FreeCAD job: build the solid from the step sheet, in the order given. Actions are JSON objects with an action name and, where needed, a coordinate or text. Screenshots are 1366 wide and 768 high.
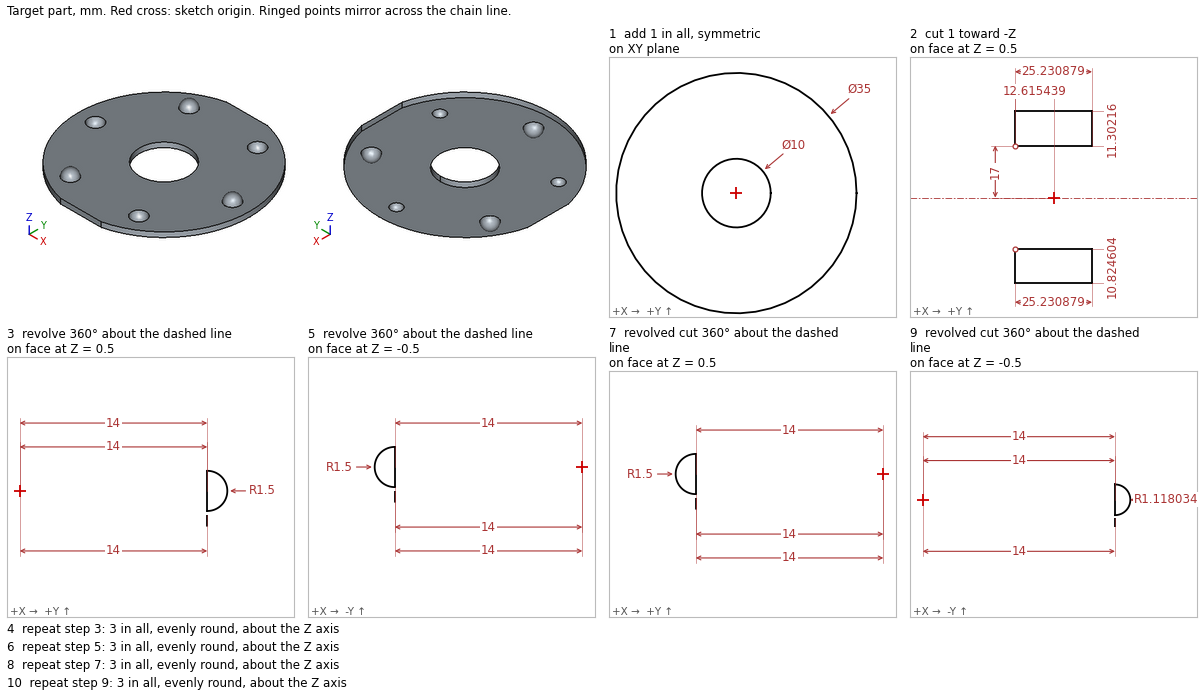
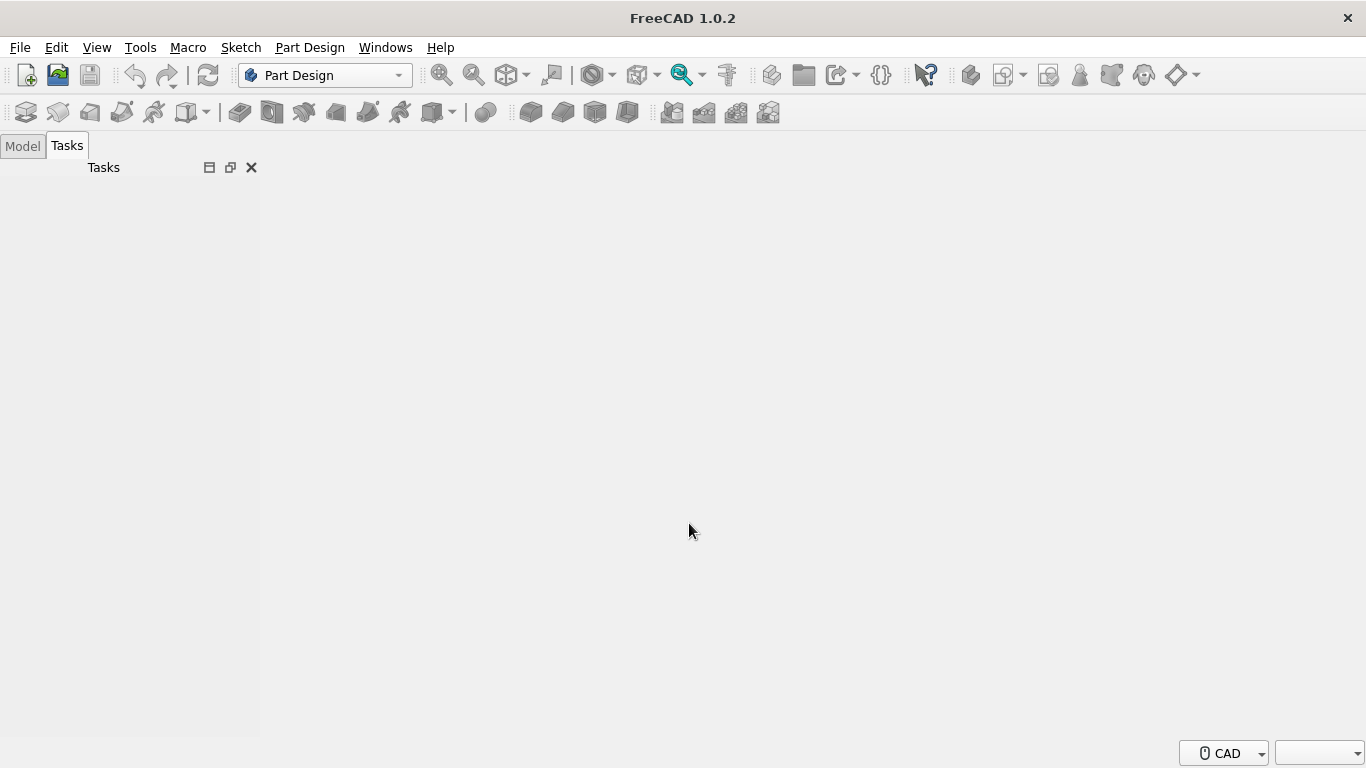
{"action": "key", "text": "ctrl+n"}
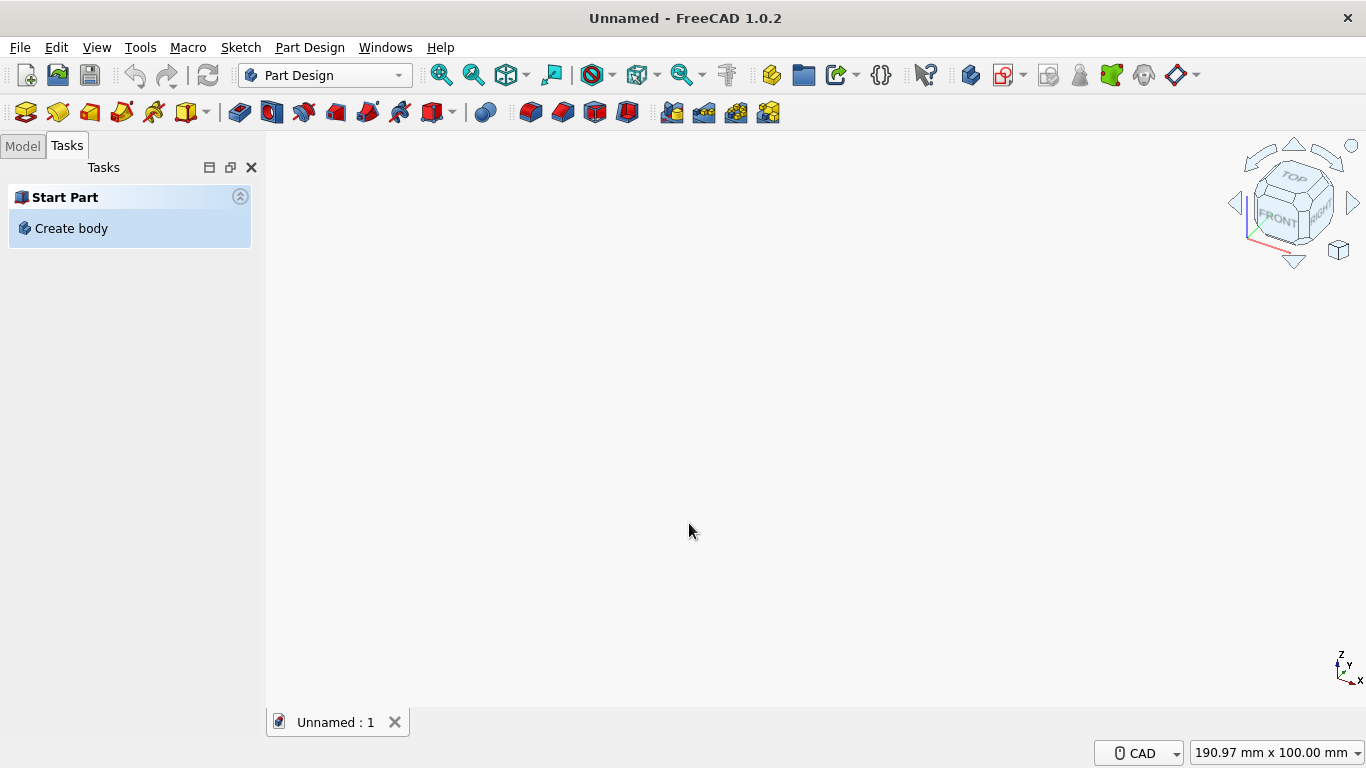
{"action": "left_click", "coordinate": [1004, 76]}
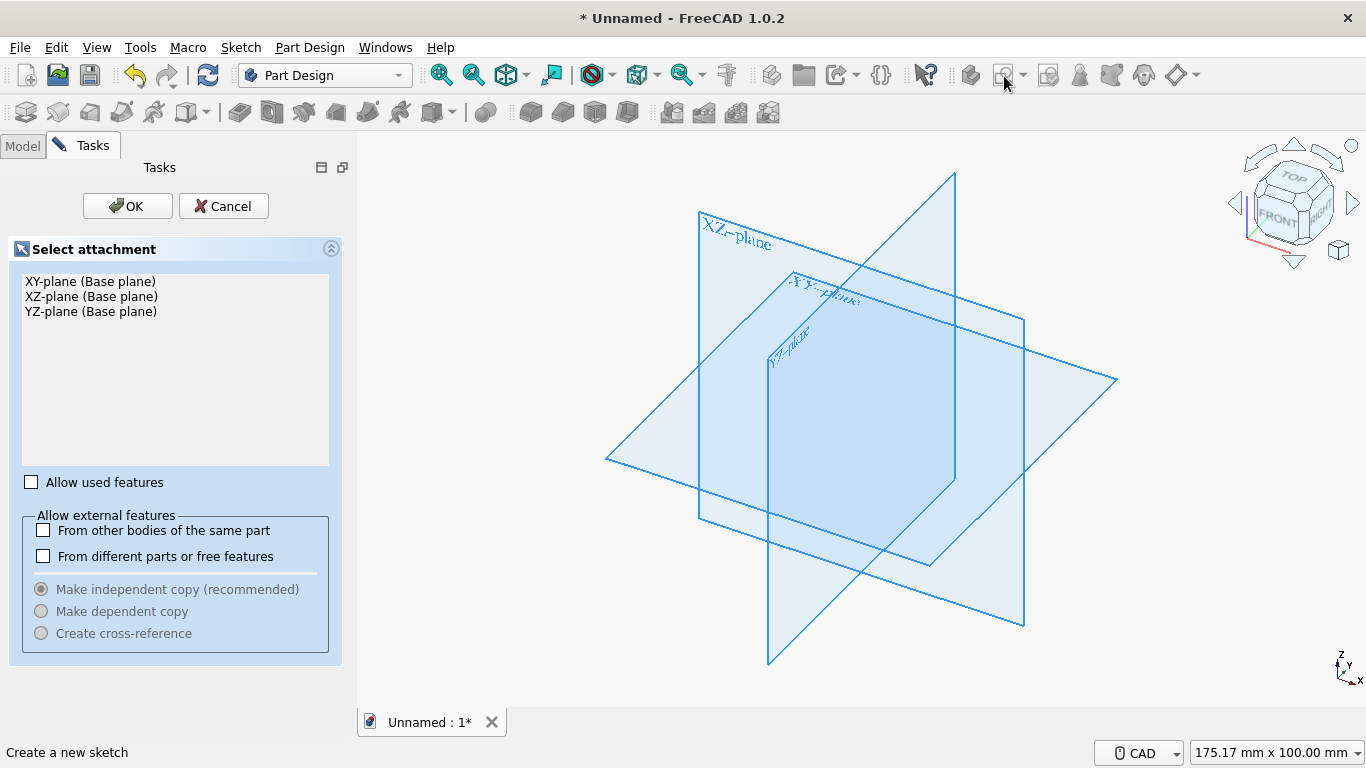
{"action": "left_click", "coordinate": [82, 282]}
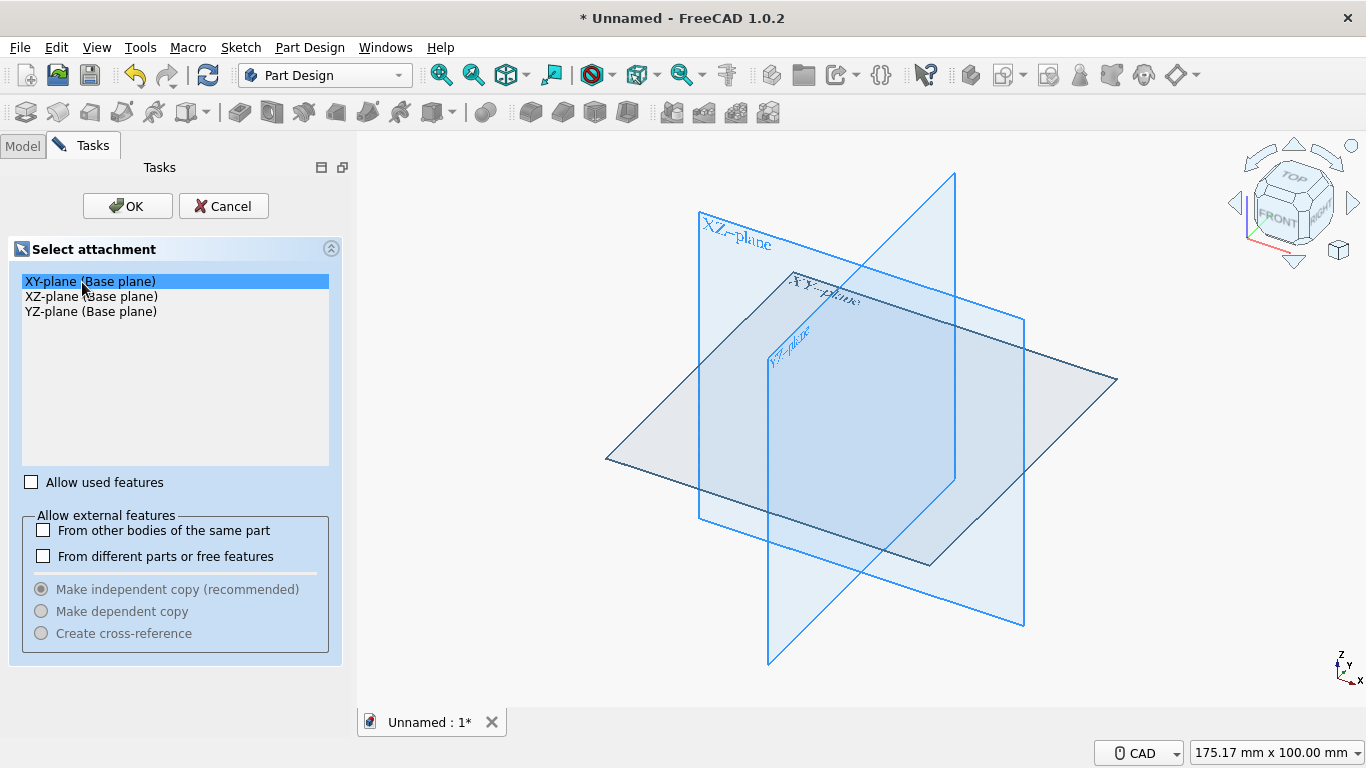
{"action": "left_click", "coordinate": [128, 206]}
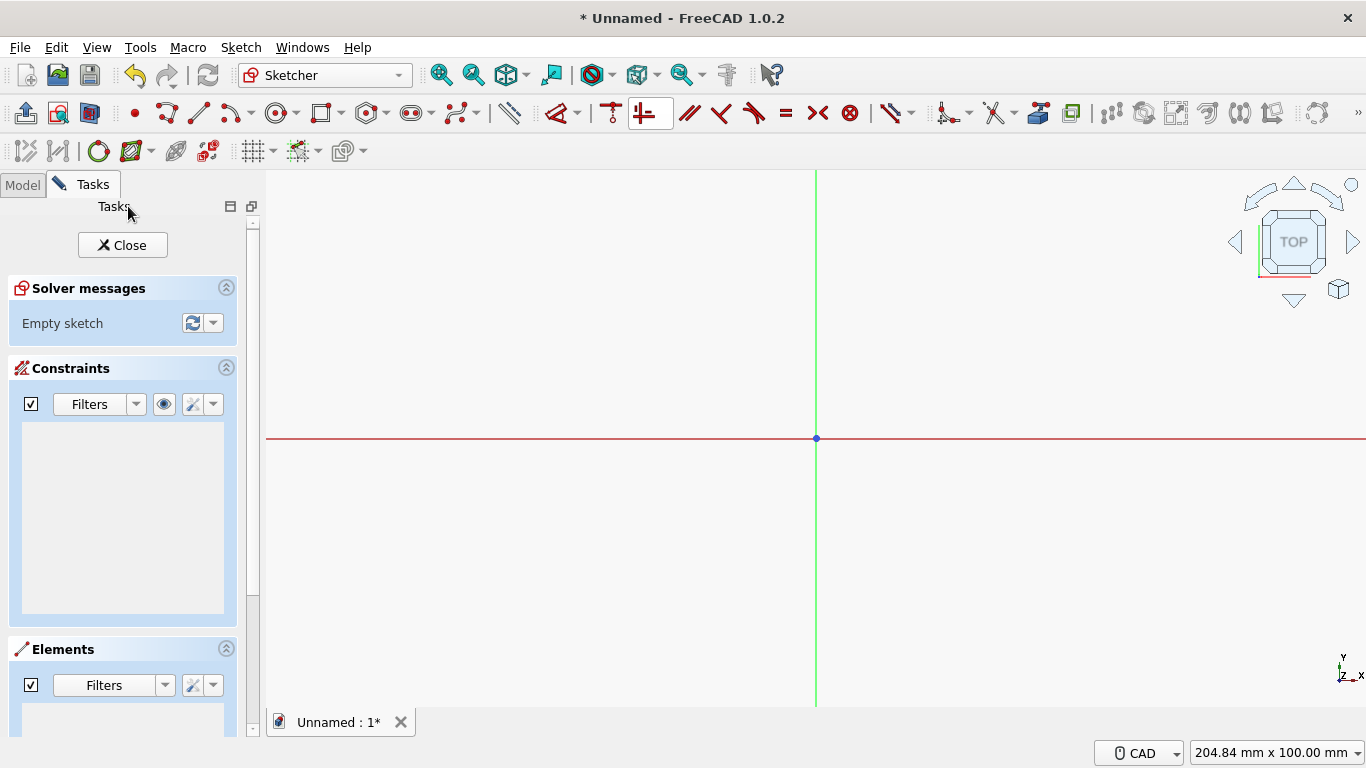
{"action": "scroll", "coordinate": [899, 438], "scroll_direction": "up", "scroll_amount": 3}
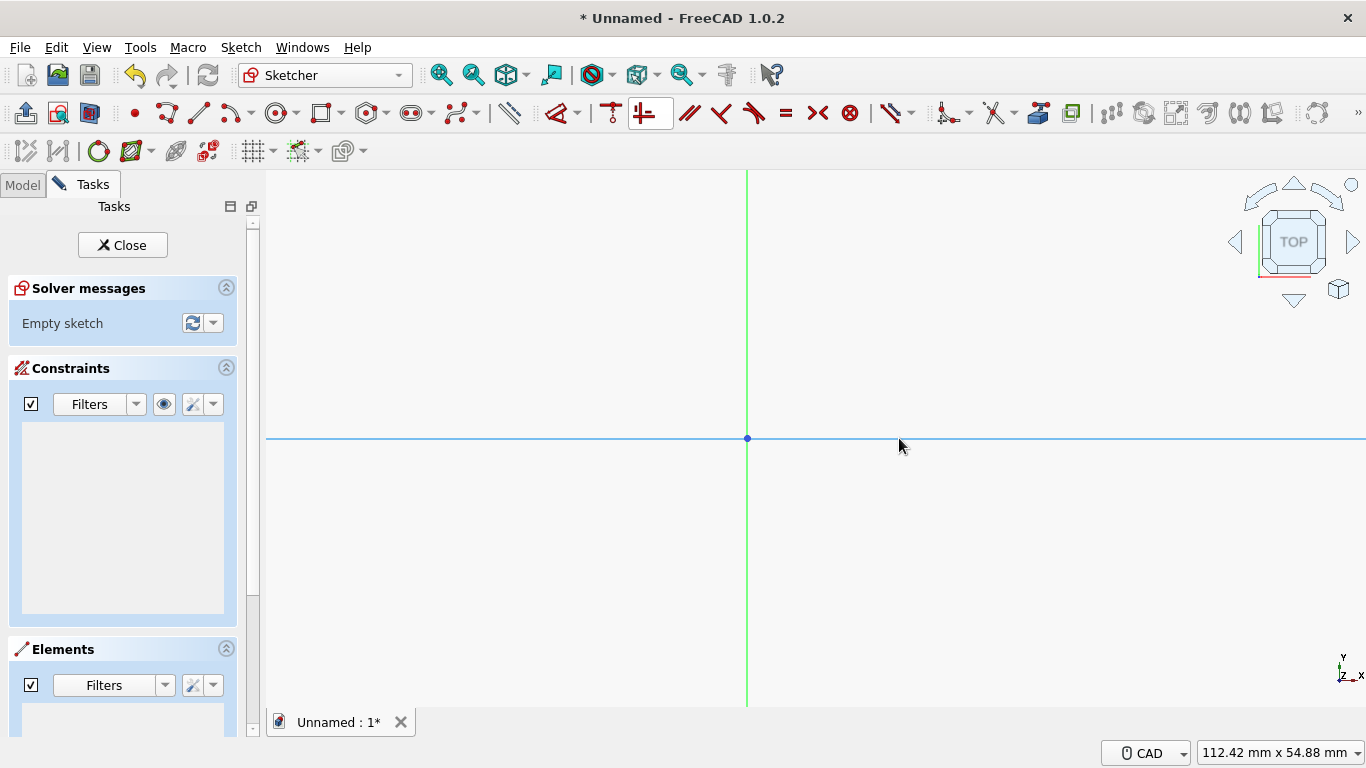
{"action": "key", "text": "g c"}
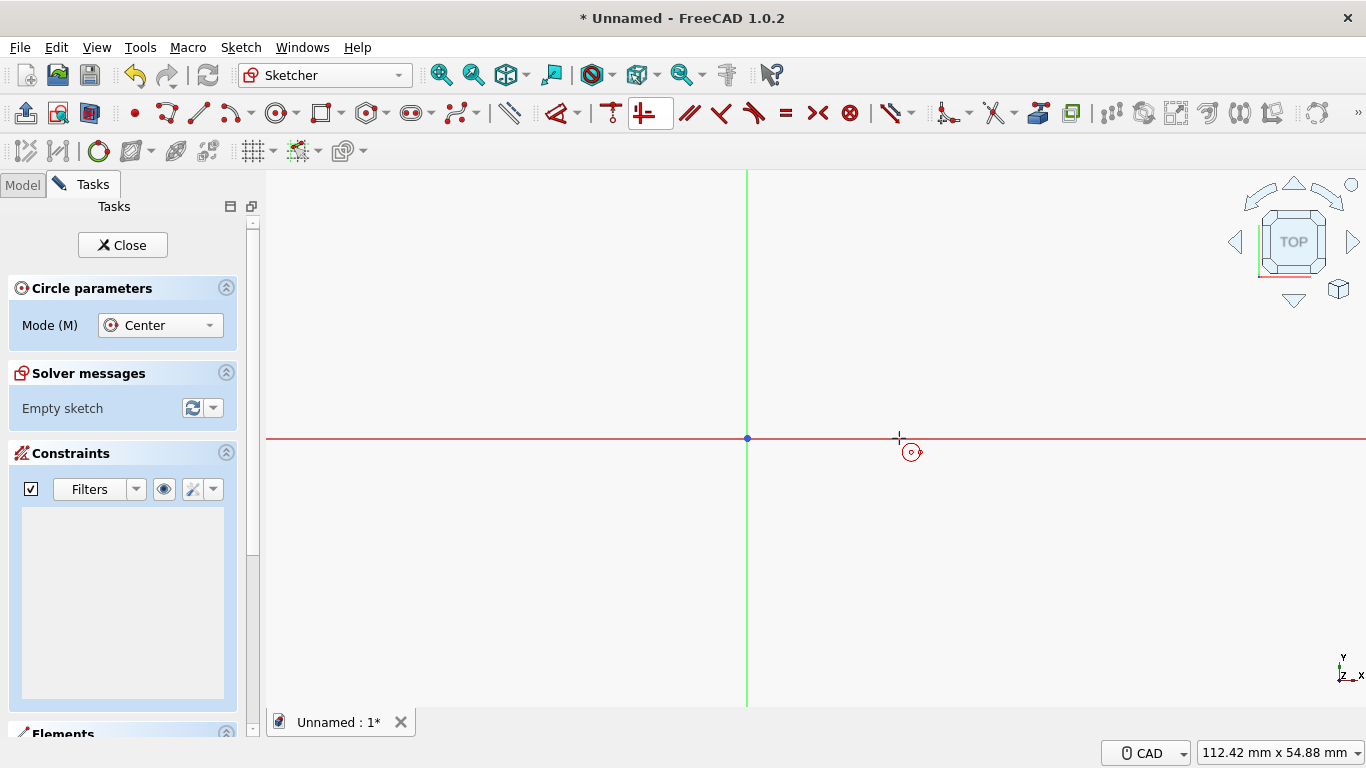
{"action": "left_click", "coordinate": [747, 438]}
{"action": "mouse_move", "coordinate": [868, 317]}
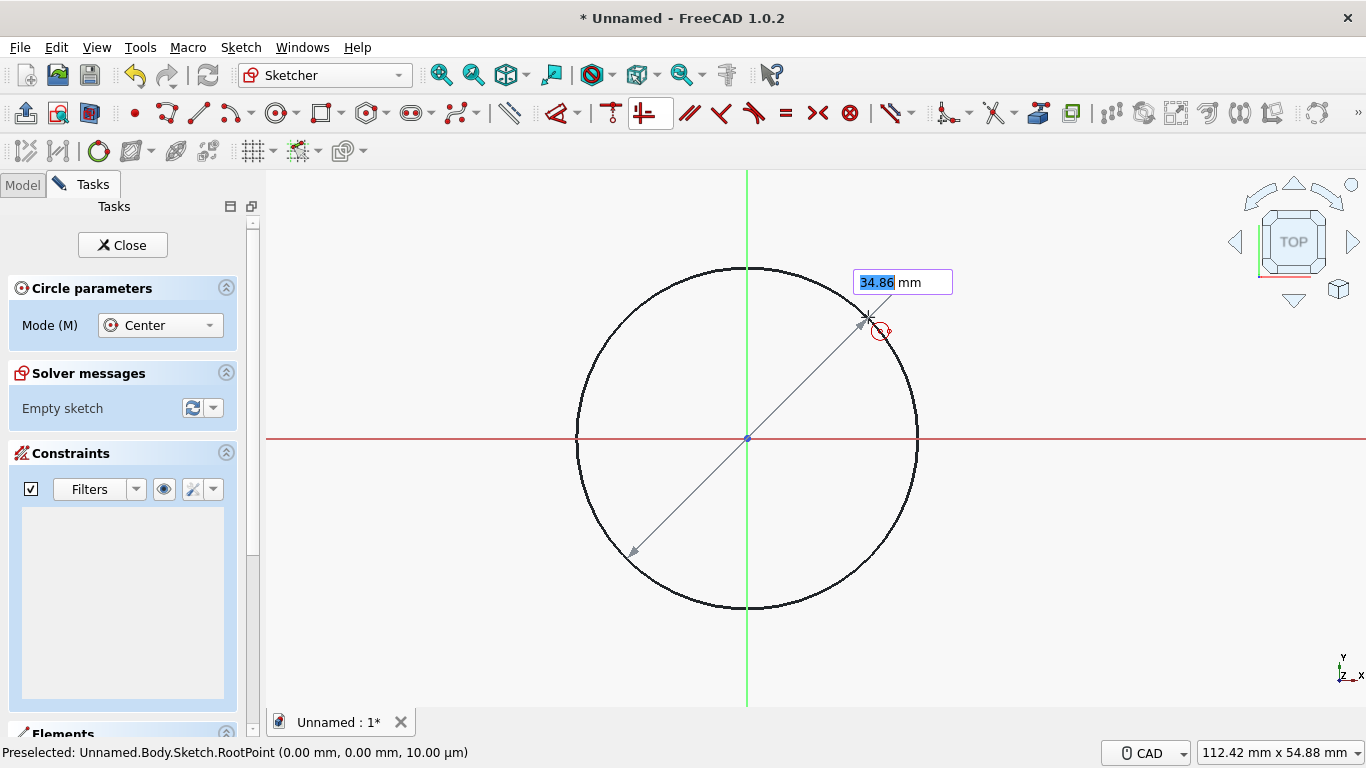
{"action": "type", "text": "35"}
{"action": "key", "text": "Return"}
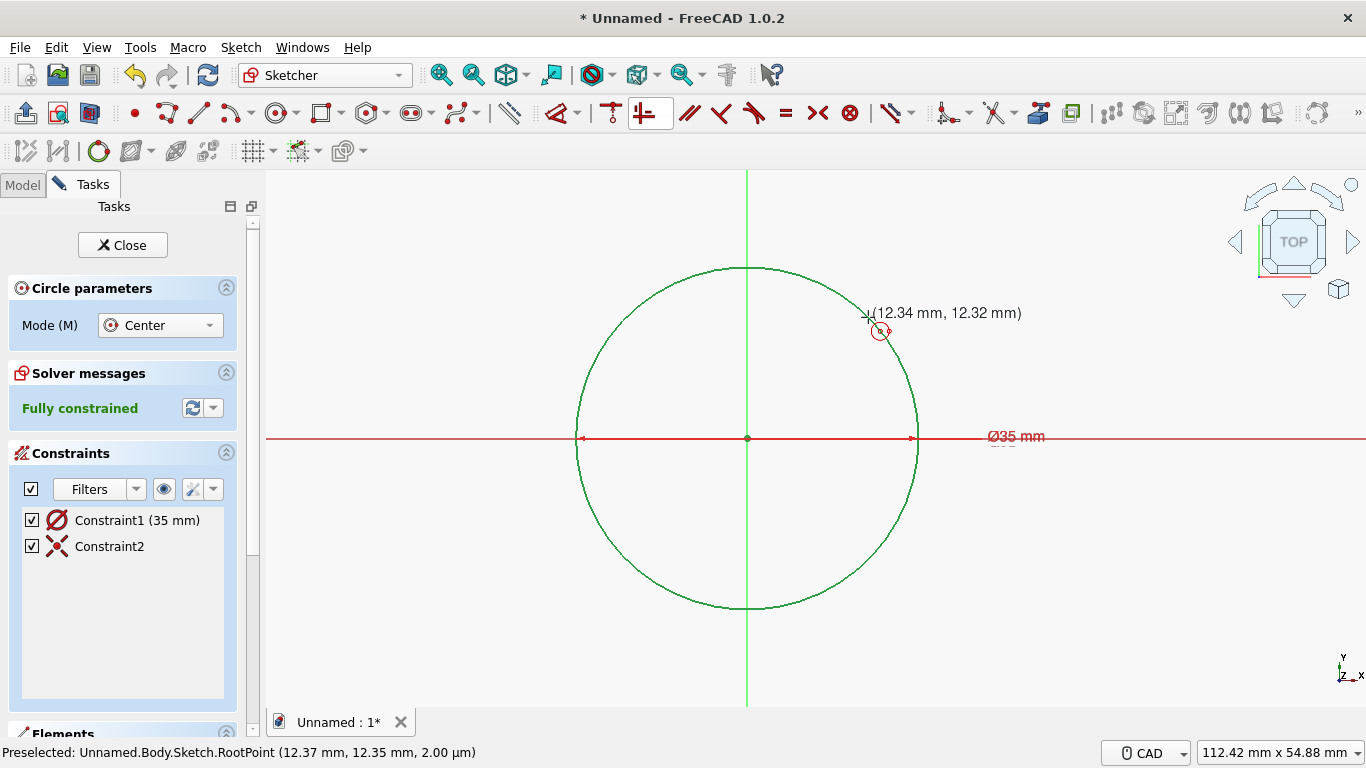
{"action": "left_click", "coordinate": [747, 438]}
{"action": "mouse_move", "coordinate": [782, 404]}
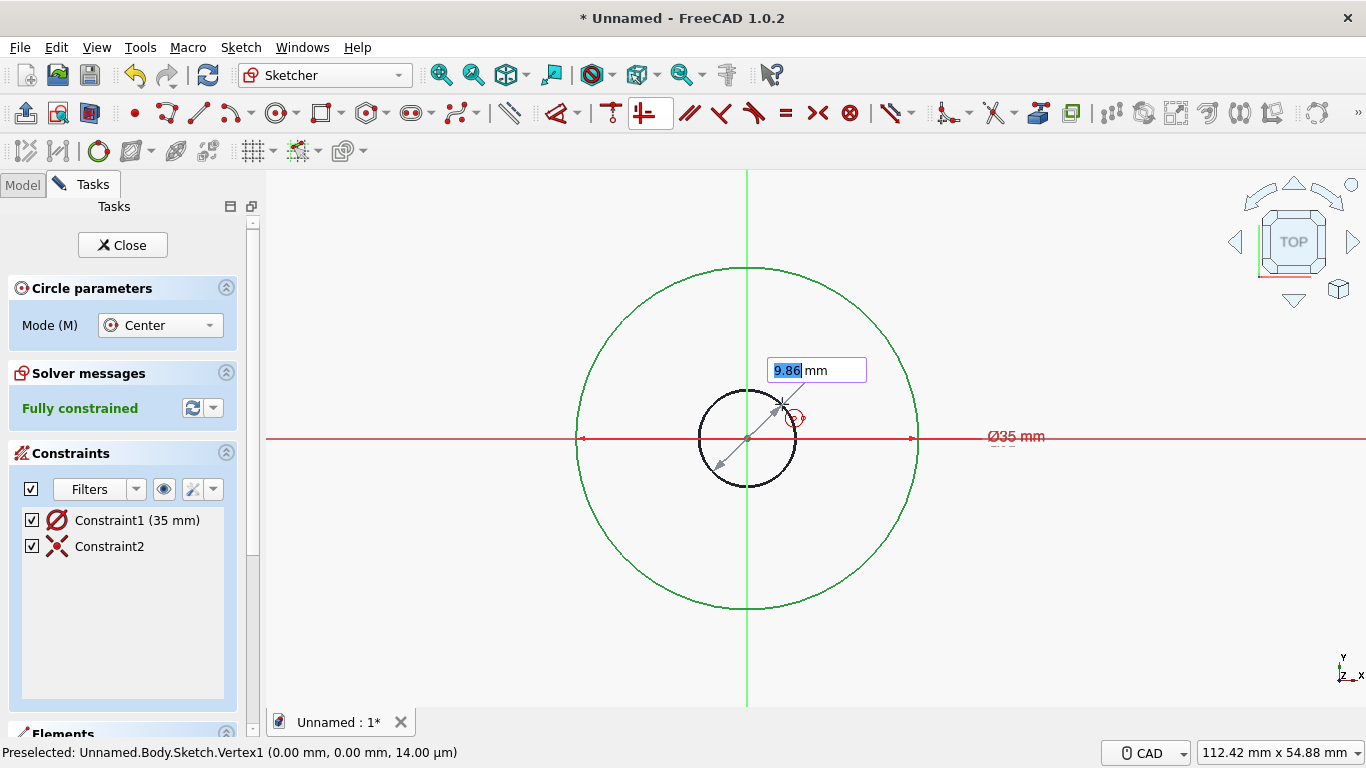
{"action": "type", "text": "10"}
{"action": "key", "text": "Return"}
{"action": "key", "text": "Escape"}